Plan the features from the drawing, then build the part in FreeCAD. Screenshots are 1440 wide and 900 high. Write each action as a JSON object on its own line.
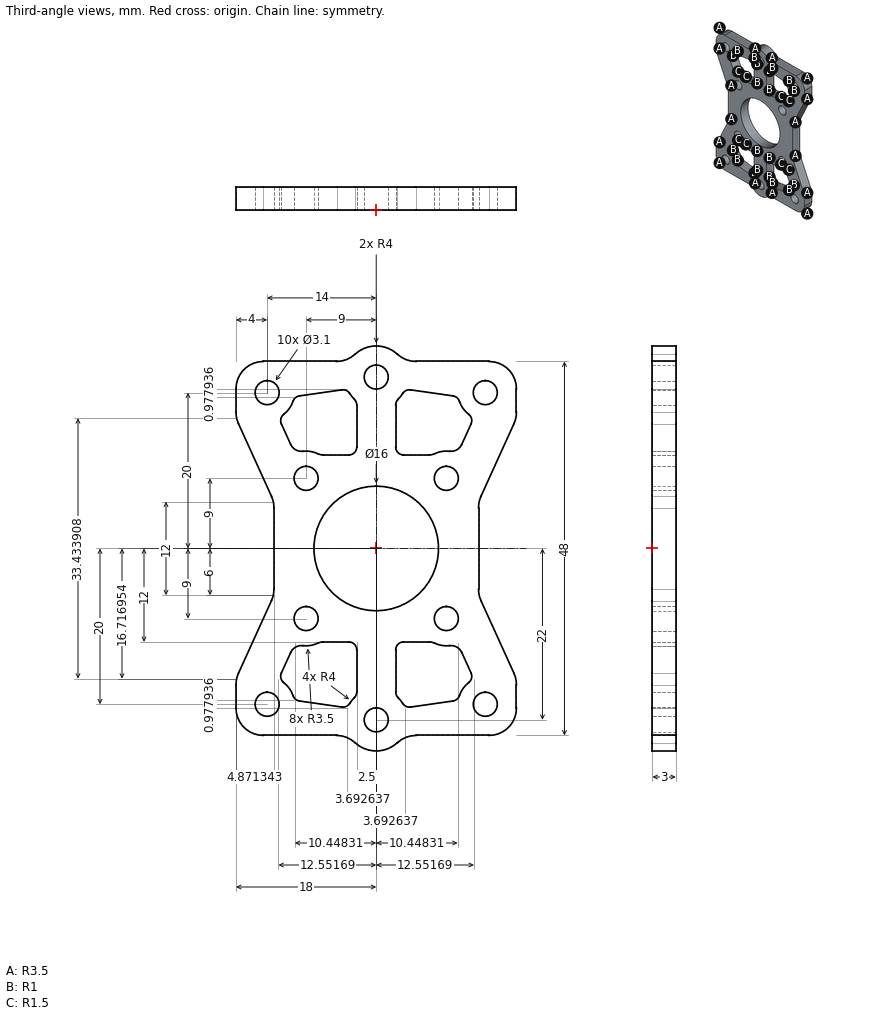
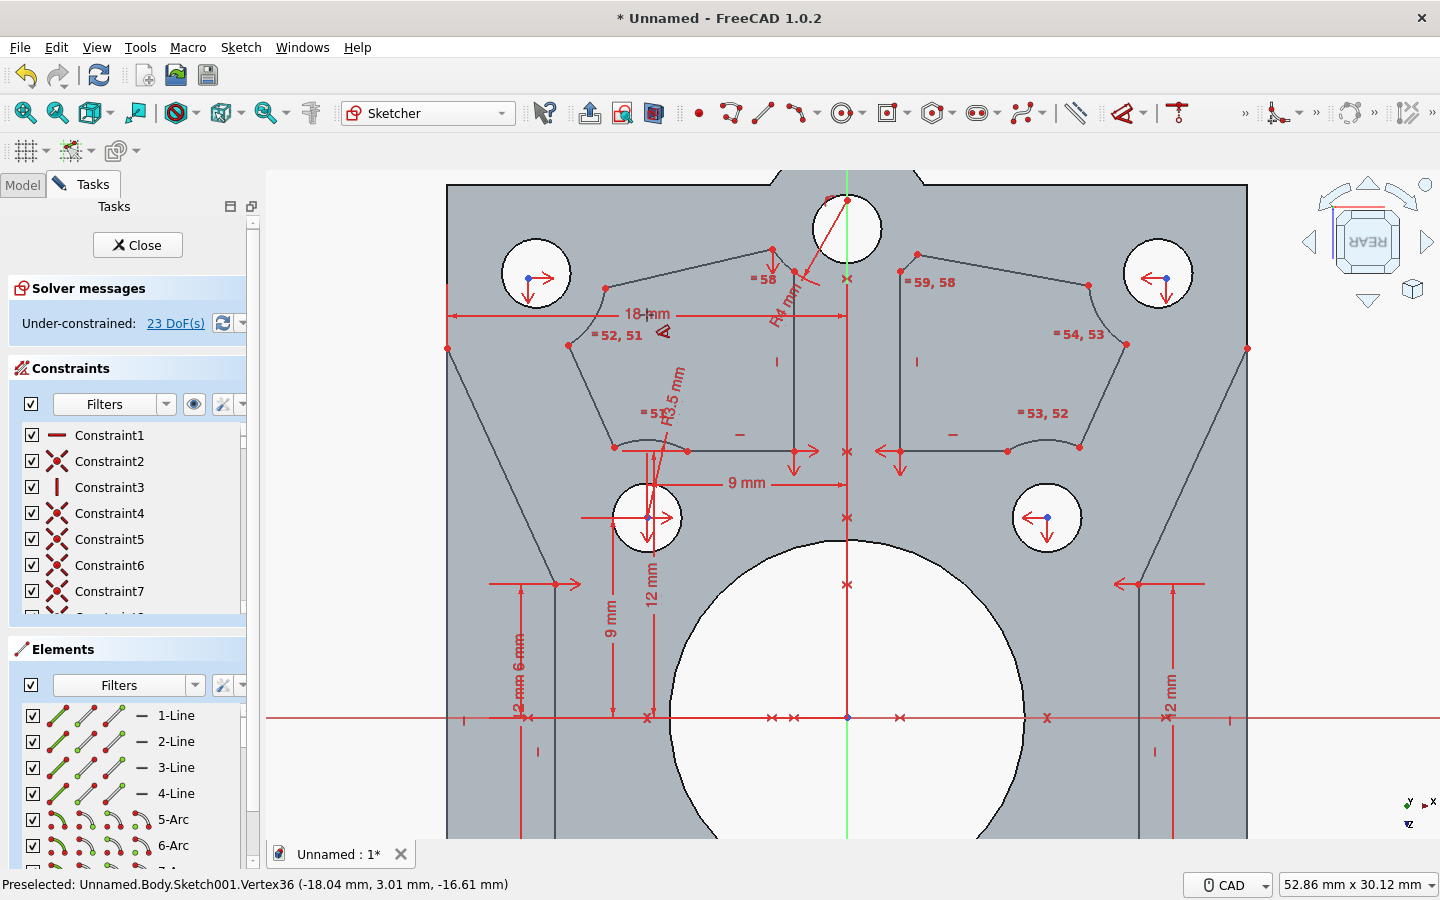
{"action": "left_click", "coordinate": [847, 201]}
{"action": "left_click", "coordinate": [881, 459]}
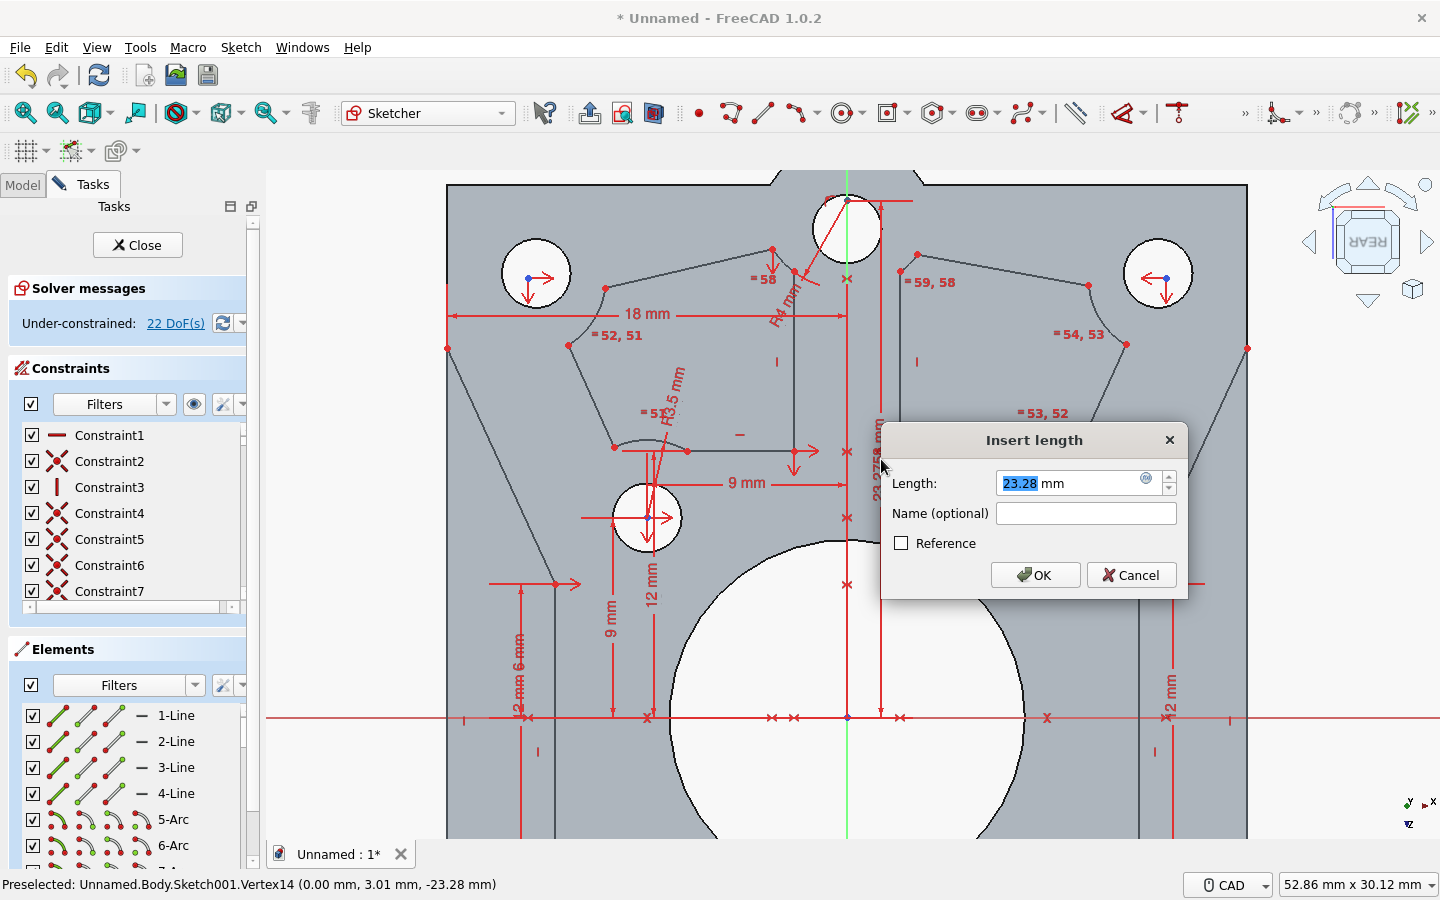
{"action": "type", "text": "22"}
{"action": "key", "text": "Return"}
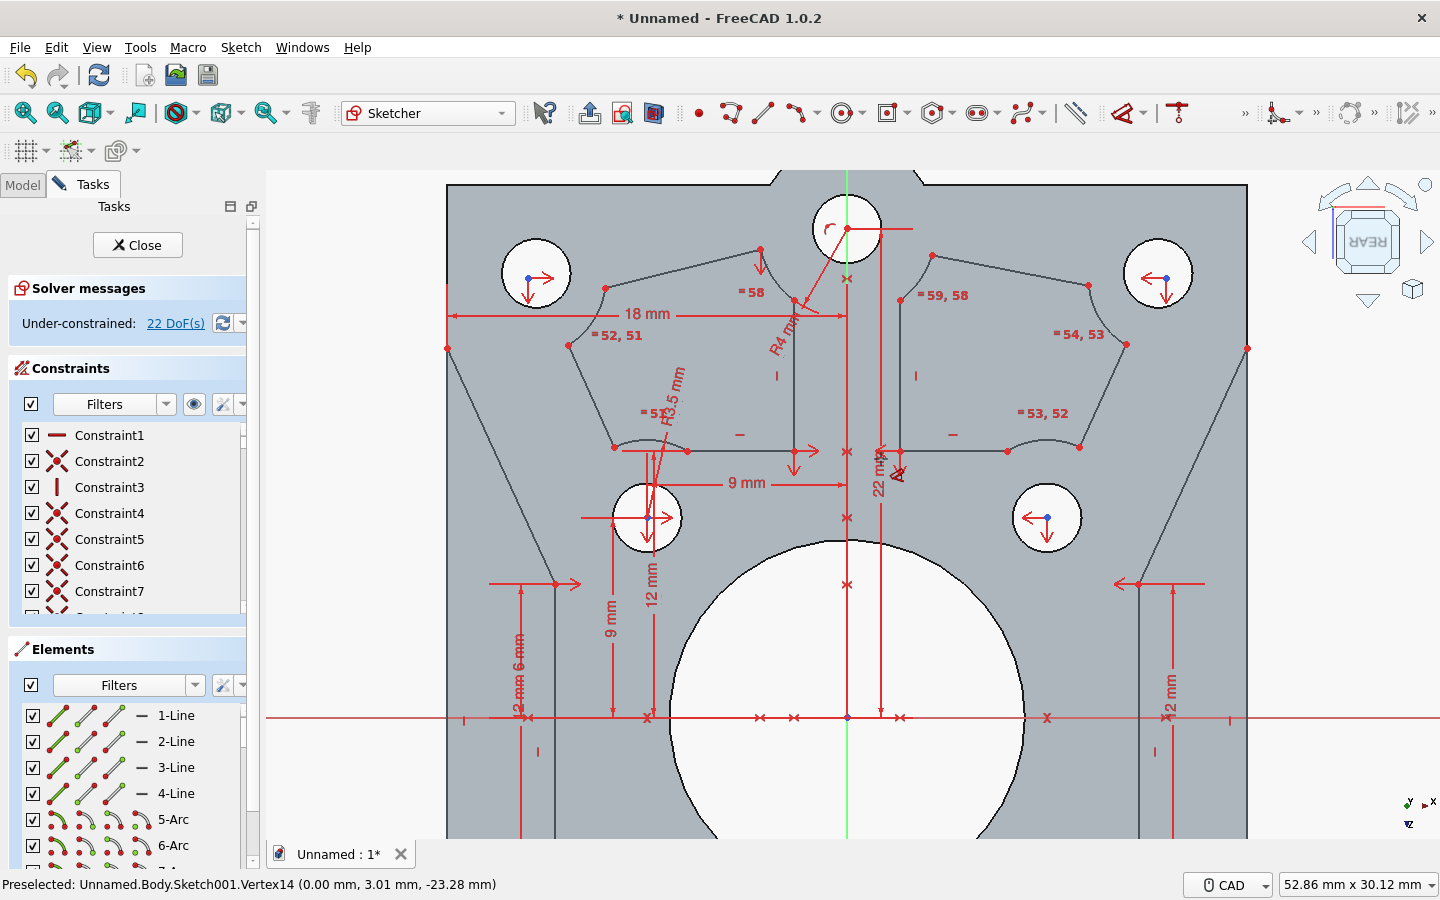
{"action": "left_click", "coordinate": [528, 278]}
{"action": "left_click", "coordinate": [688, 244]}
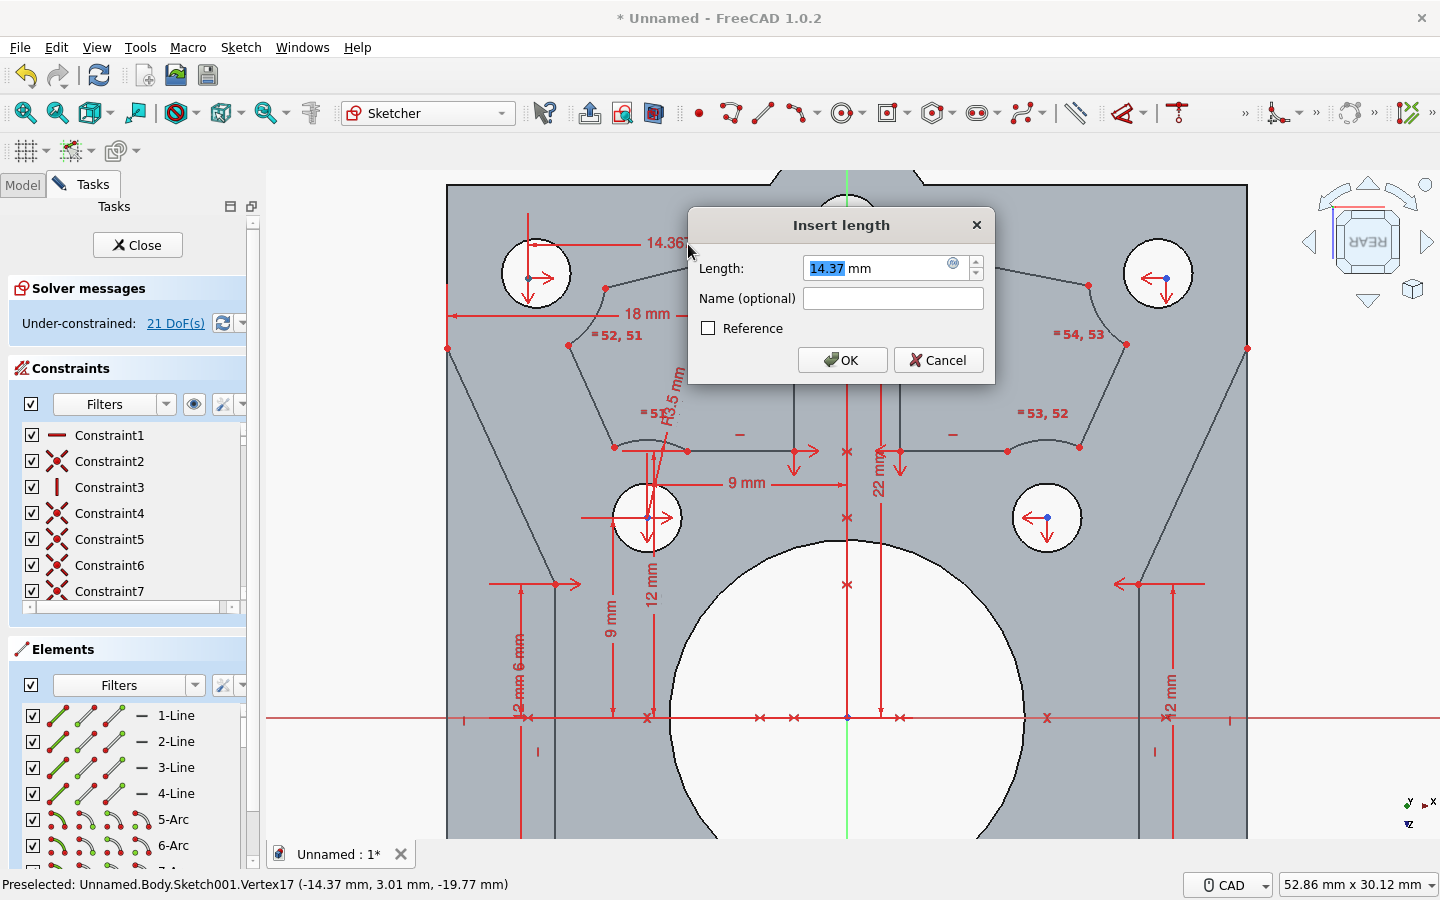
{"action": "type", "text": "14"}
{"action": "key", "text": "Return"}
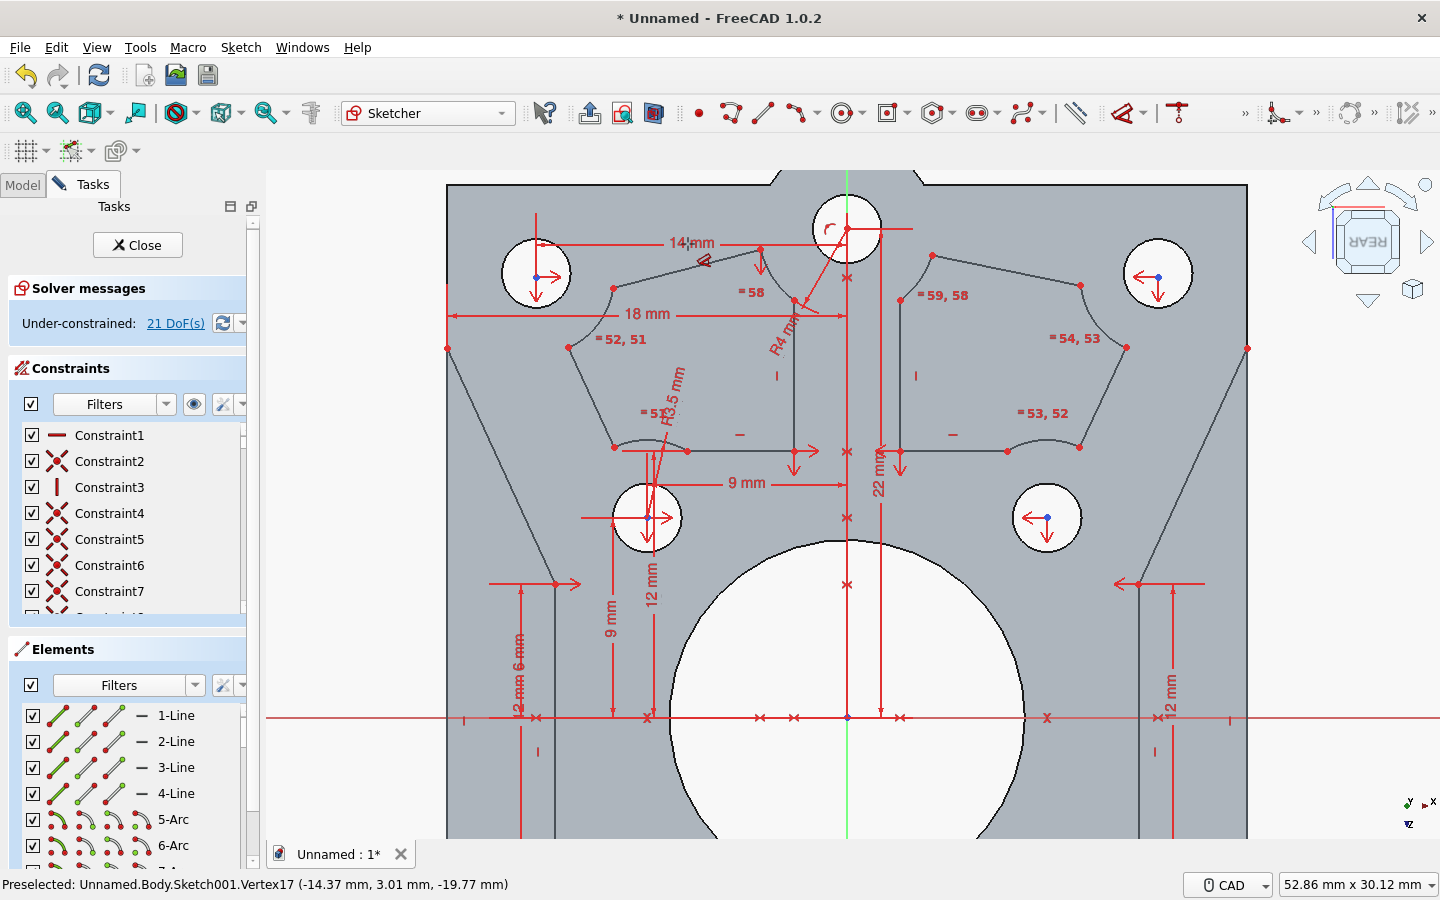
{"action": "left_click", "coordinate": [536, 277]}
{"action": "left_click", "coordinate": [502, 396]}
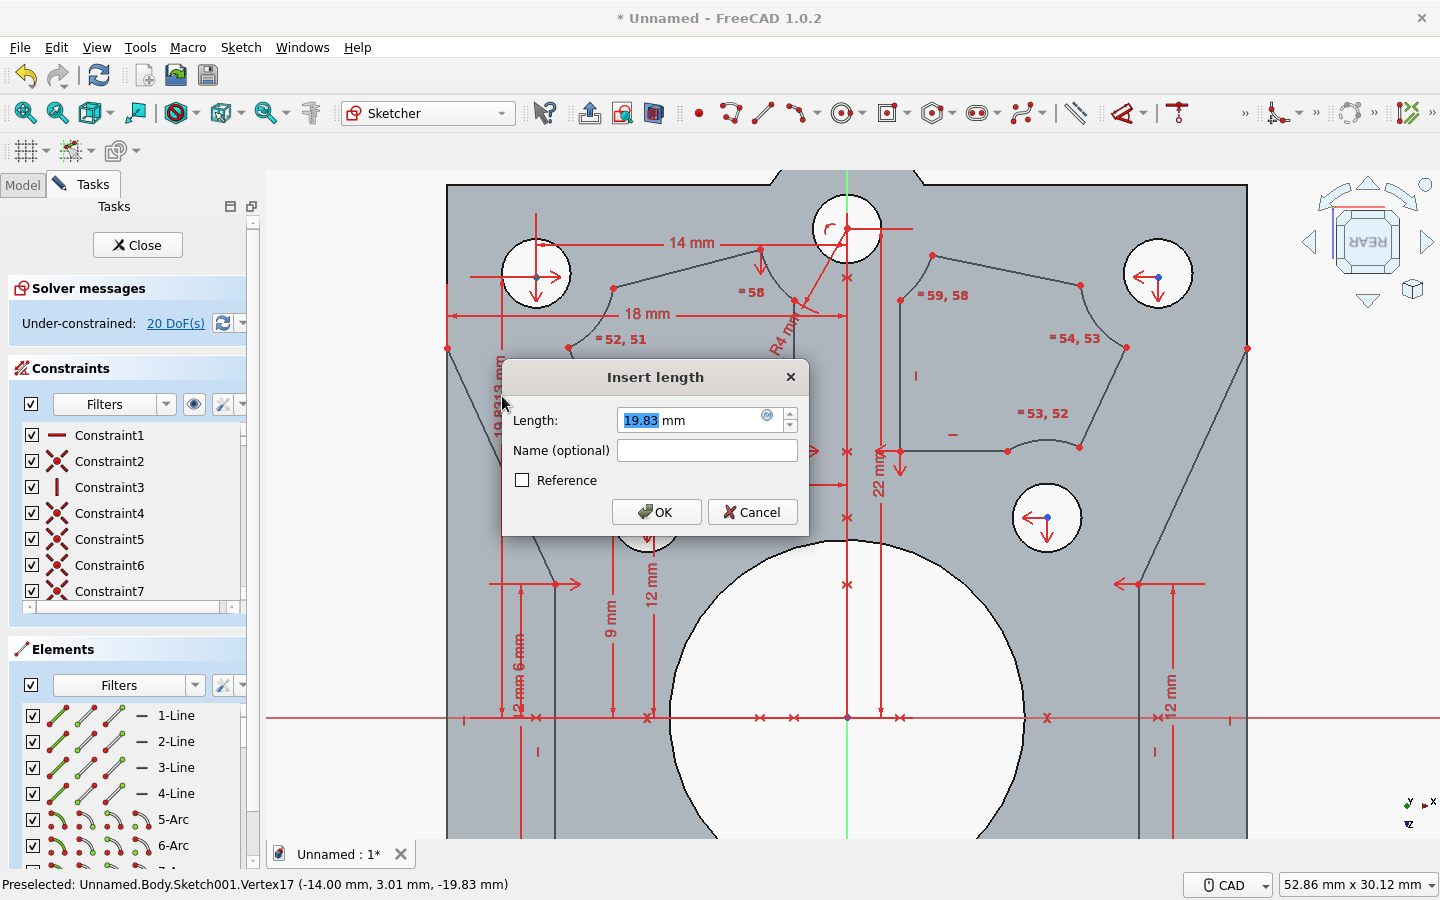
{"action": "type", "text": "20"}
{"action": "key", "text": "Return"}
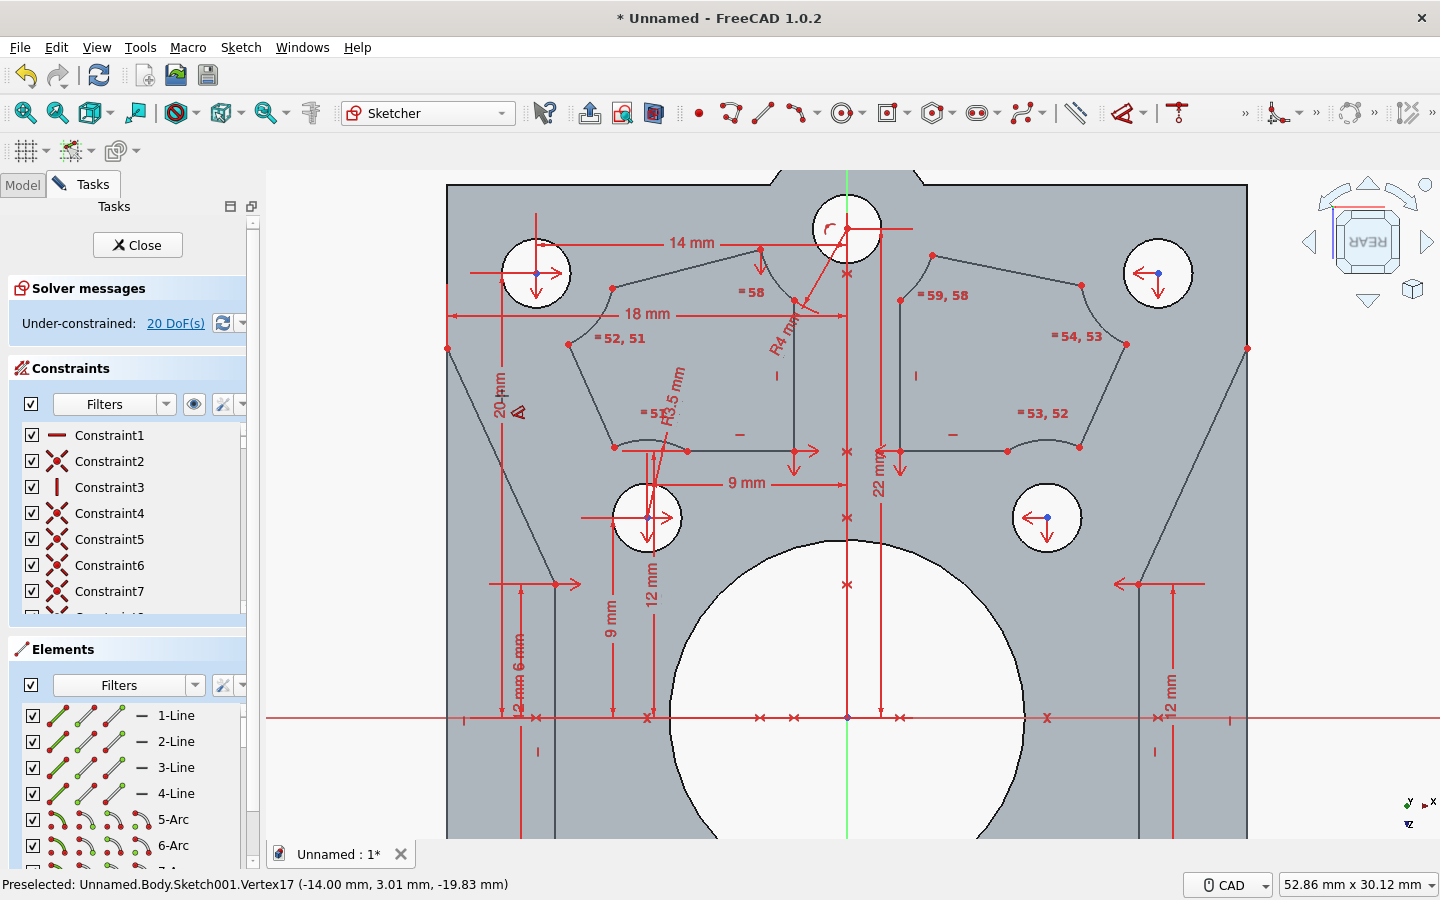
{"action": "left_click", "coordinate": [794, 451]}
{"action": "left_click", "coordinate": [821, 417]}